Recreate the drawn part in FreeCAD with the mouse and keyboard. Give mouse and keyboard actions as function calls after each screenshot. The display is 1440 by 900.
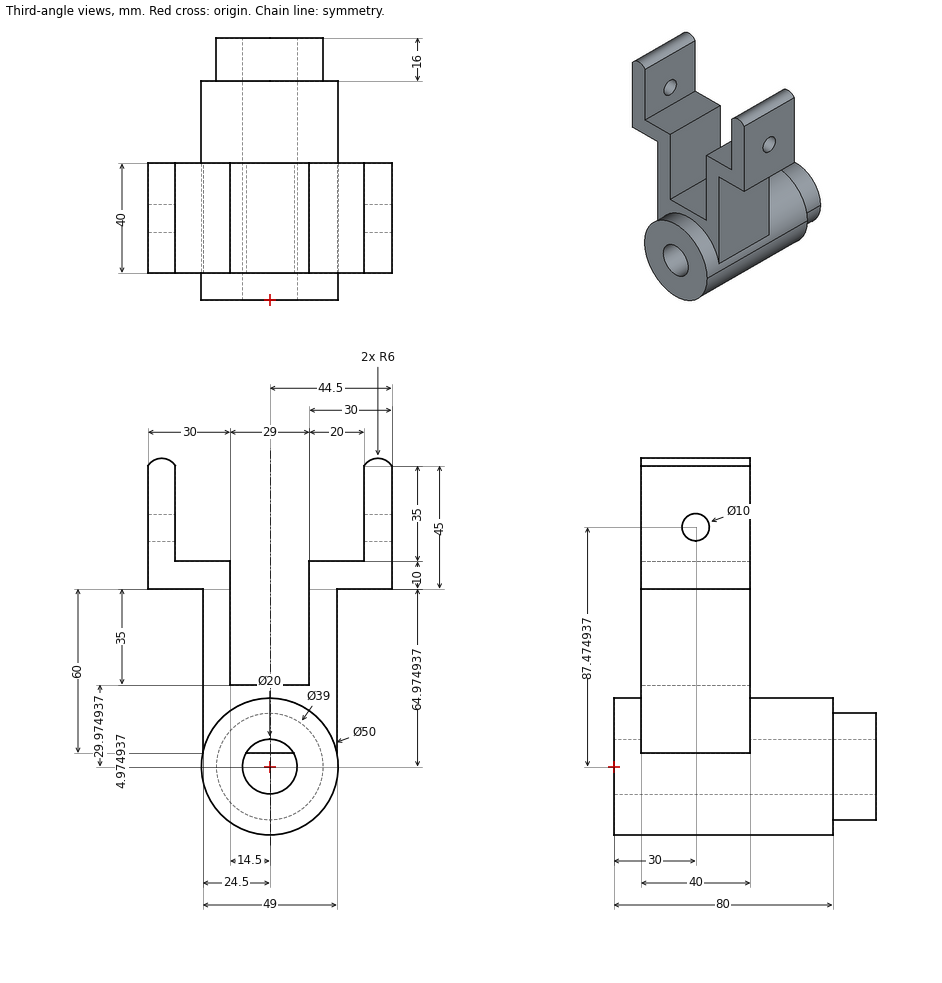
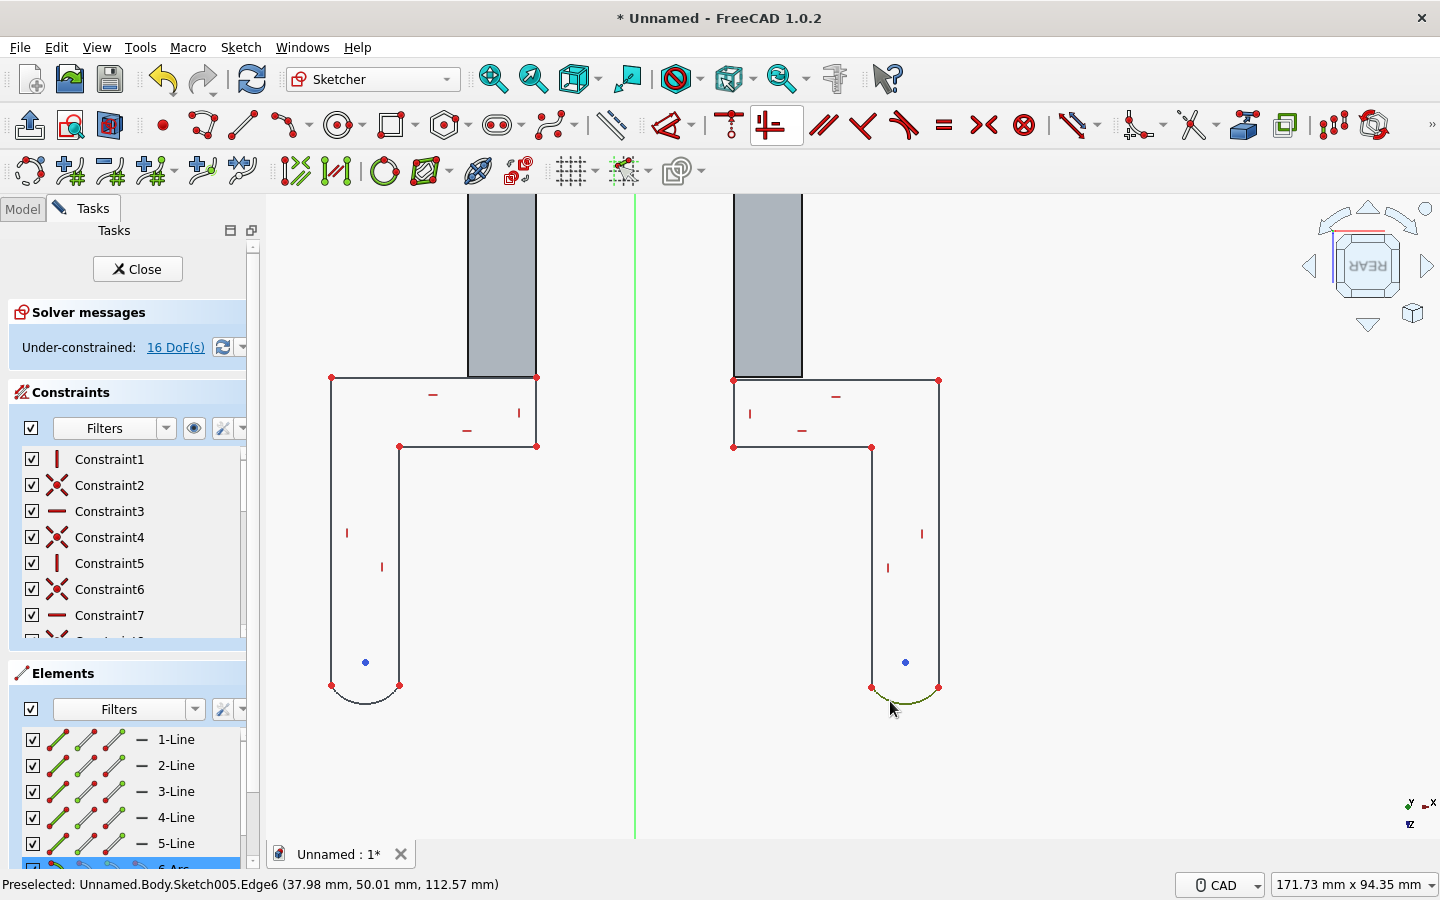
click(349, 701)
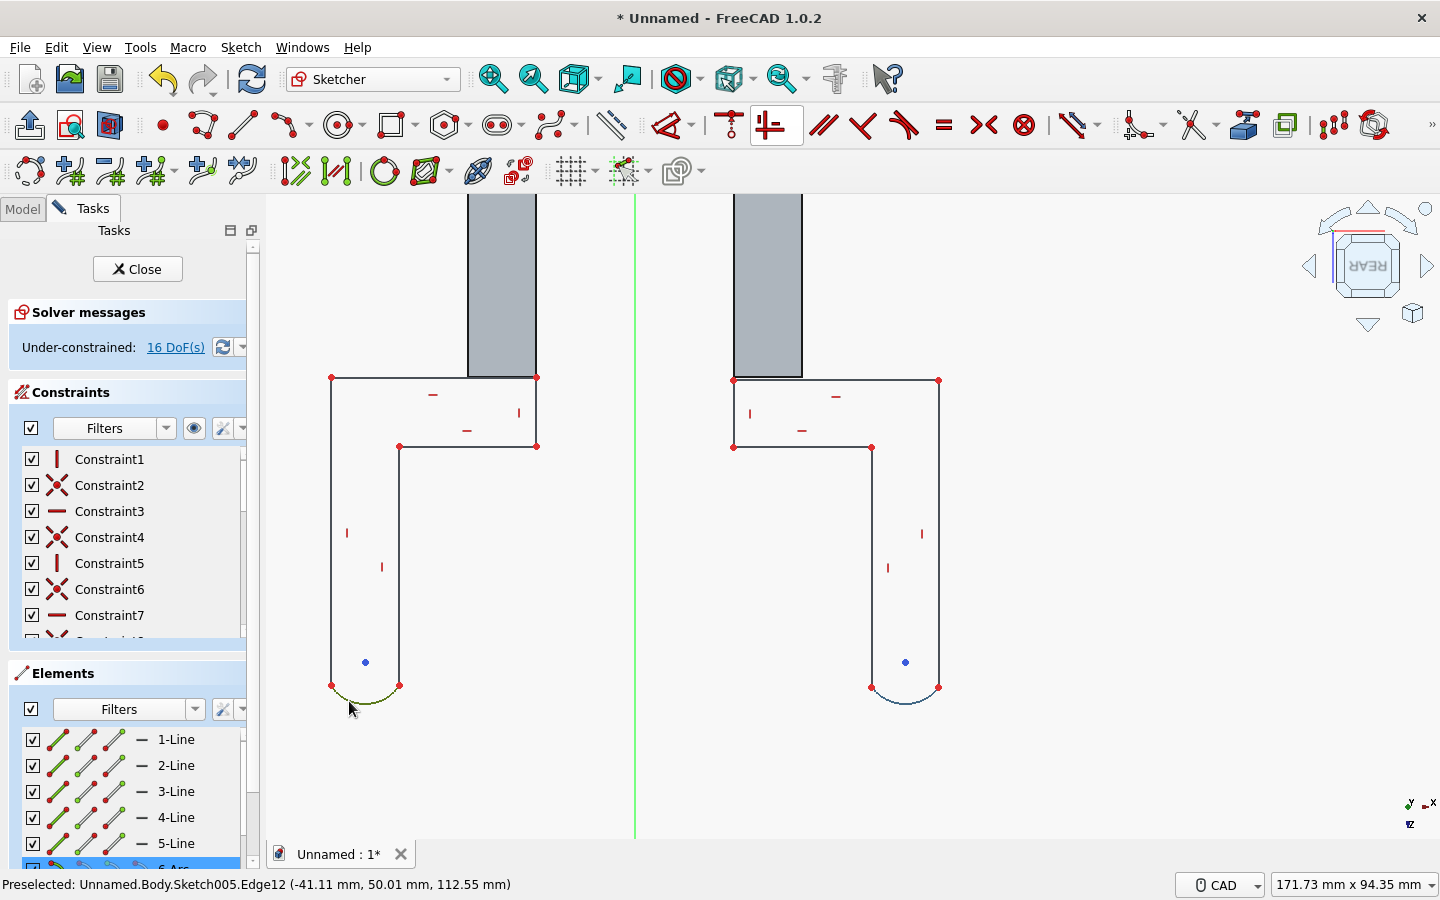
click(944, 126)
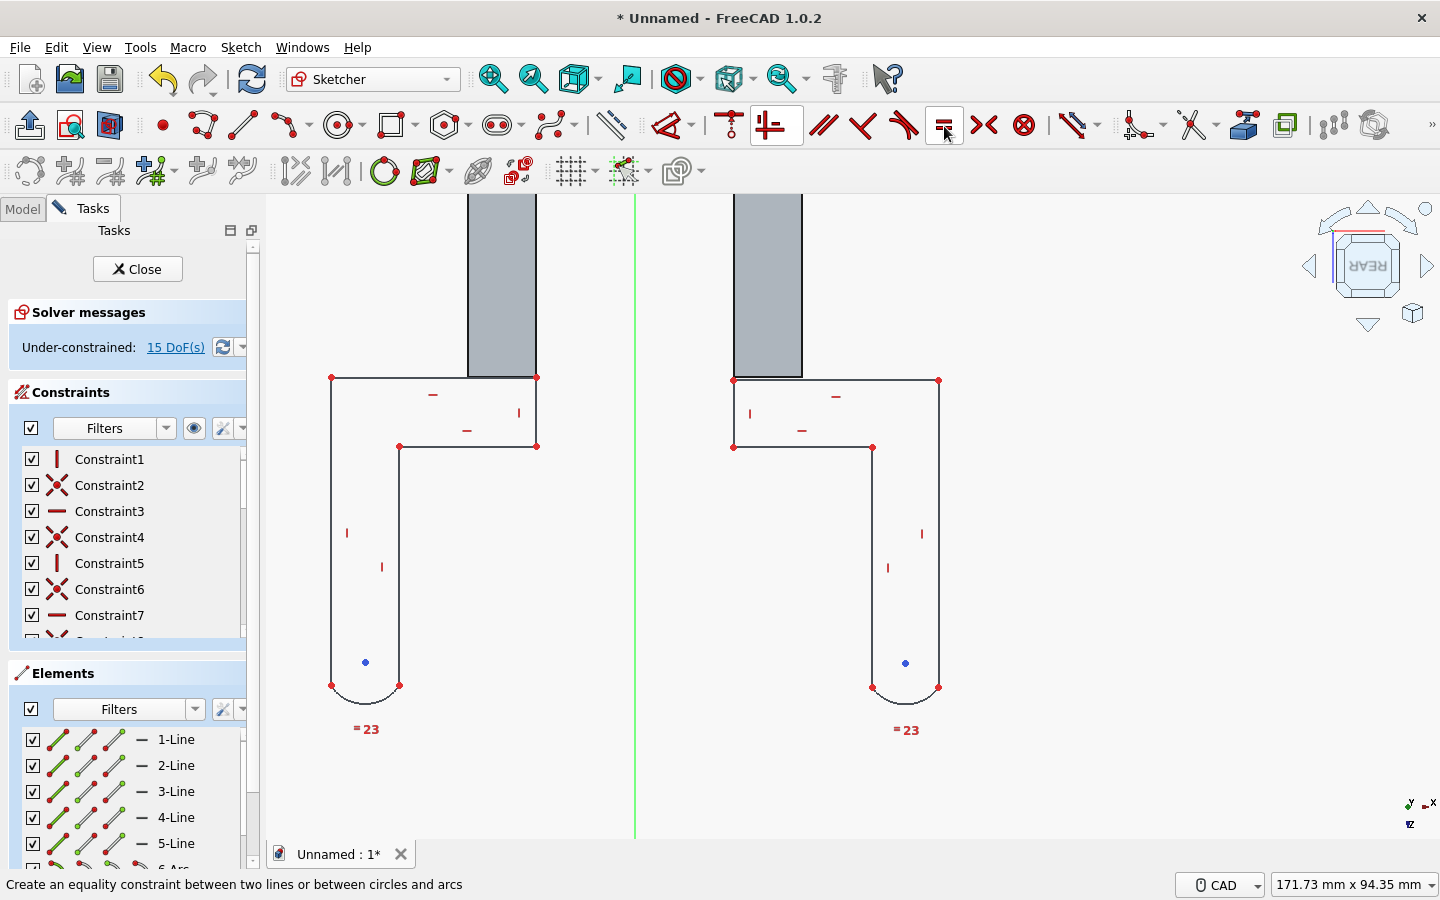
click(905, 663)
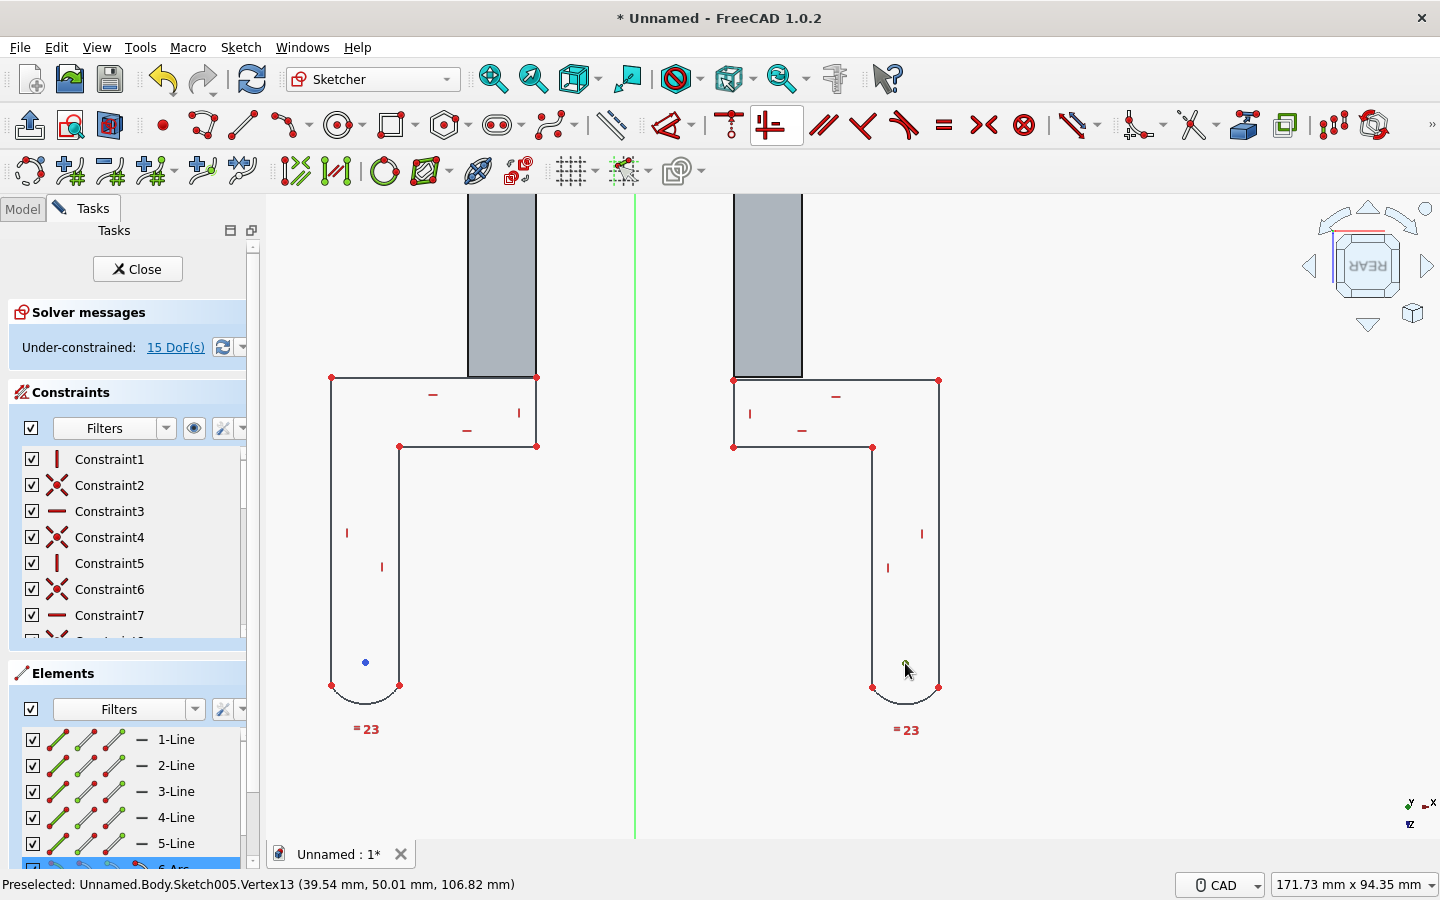
click(365, 663)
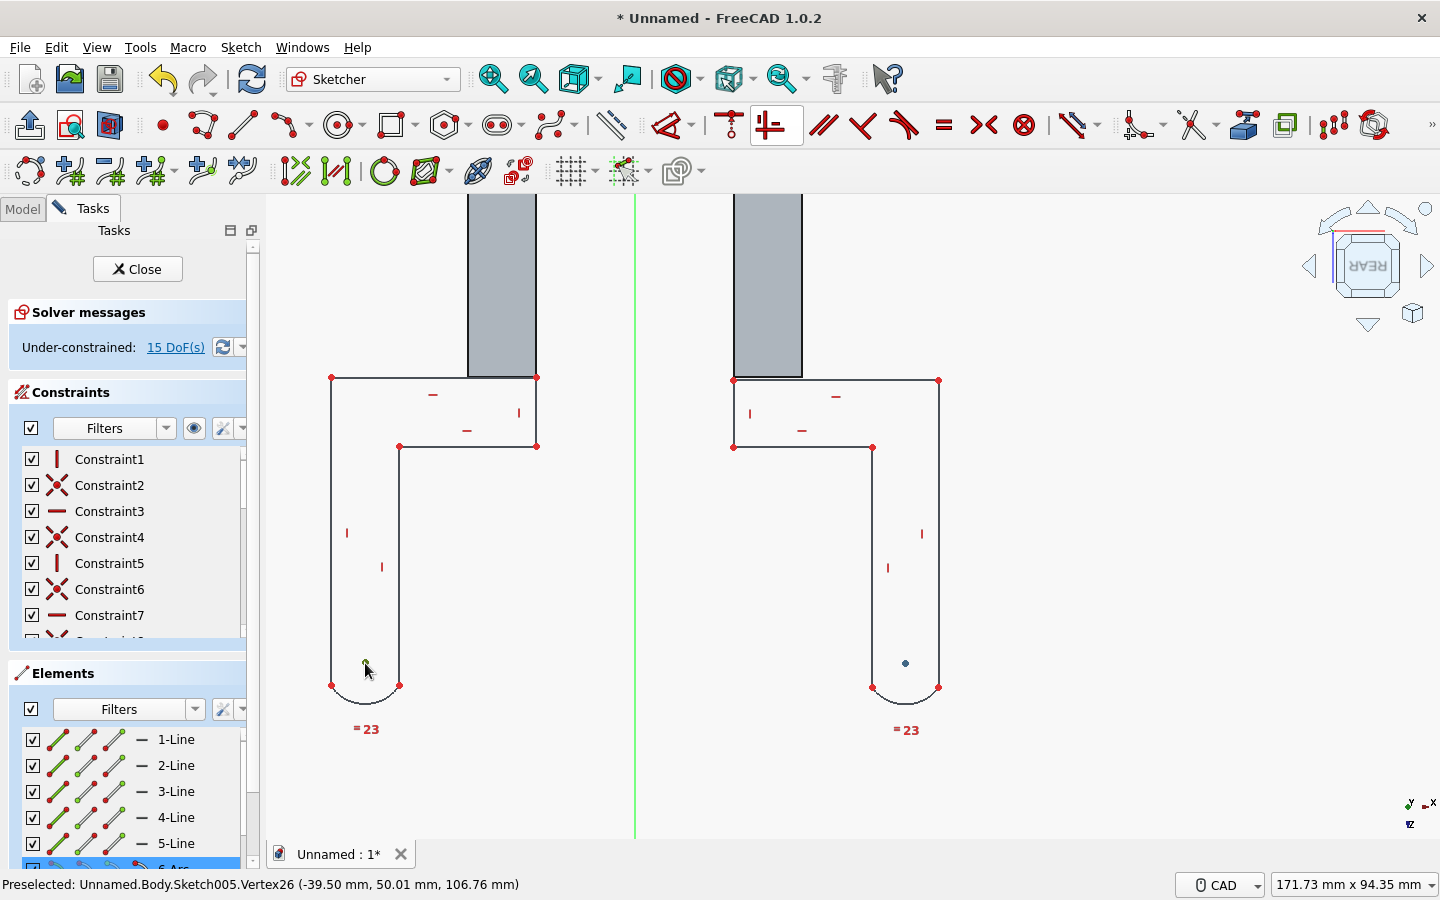
click(635, 769)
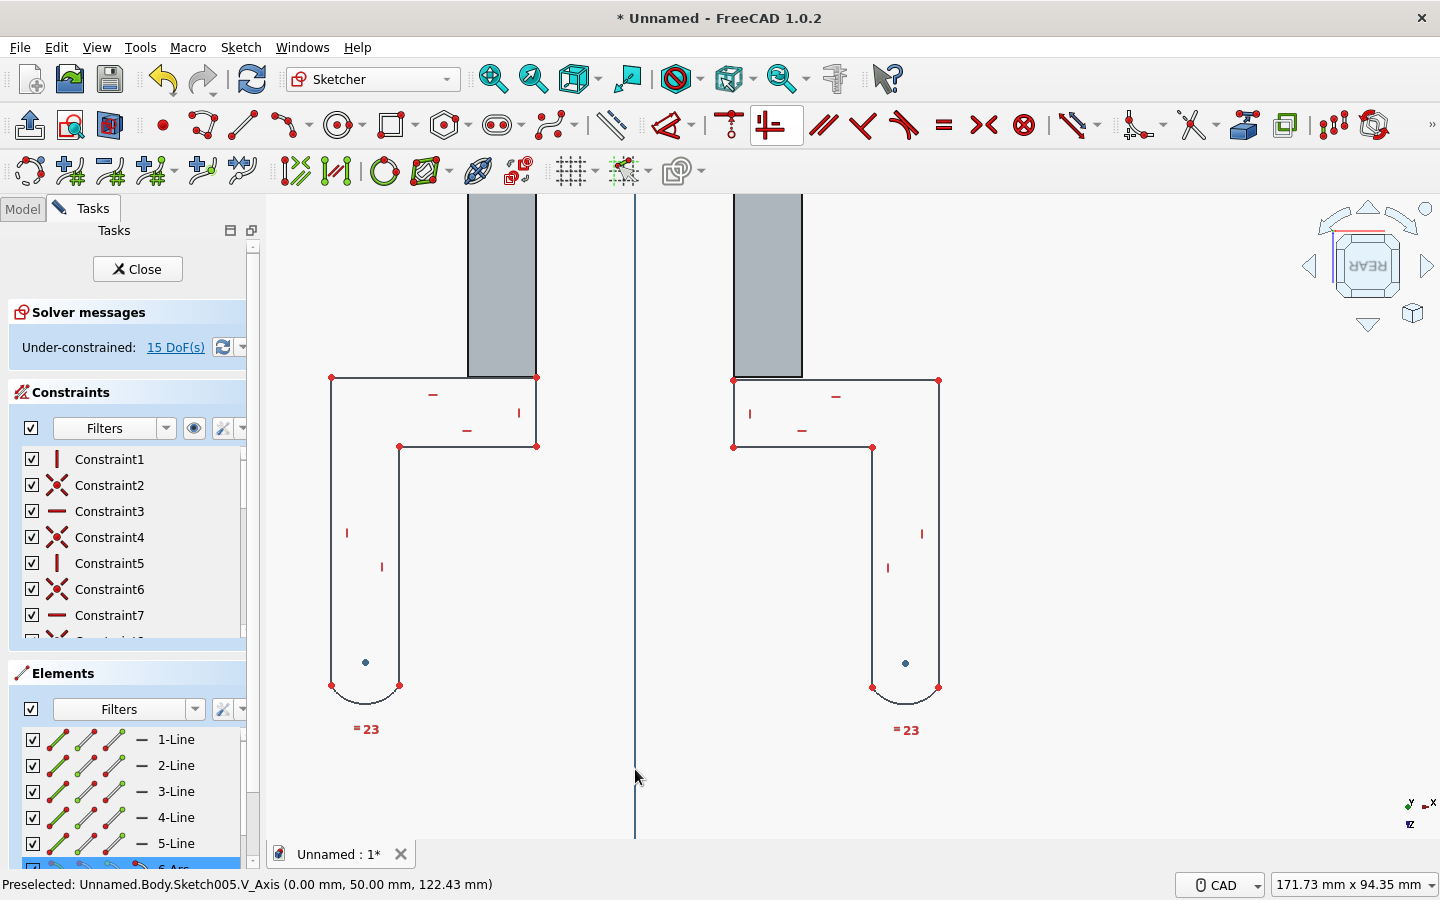
click(984, 126)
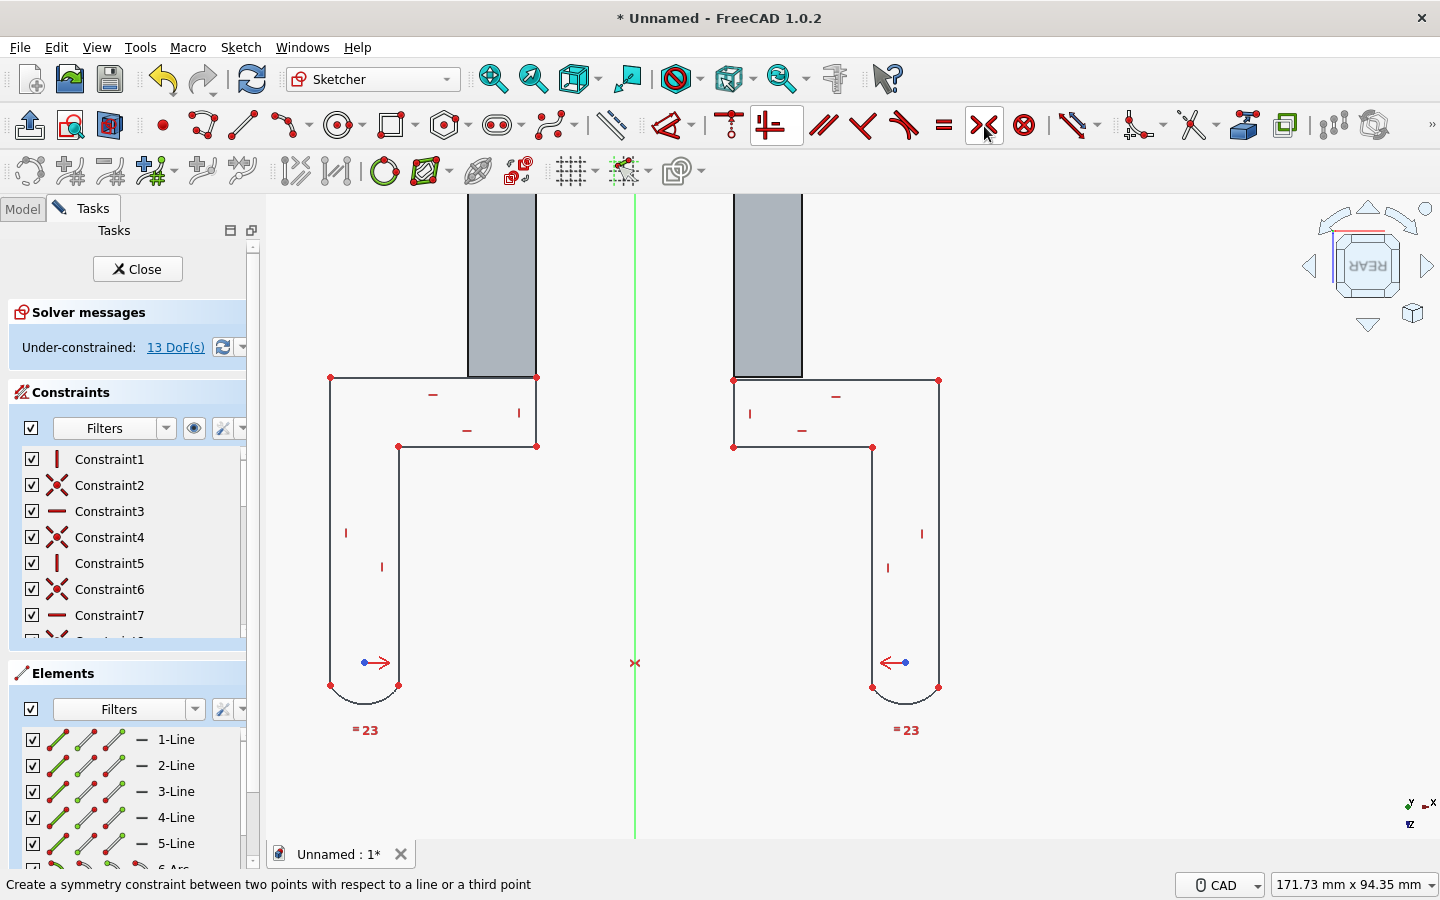
click(872, 447)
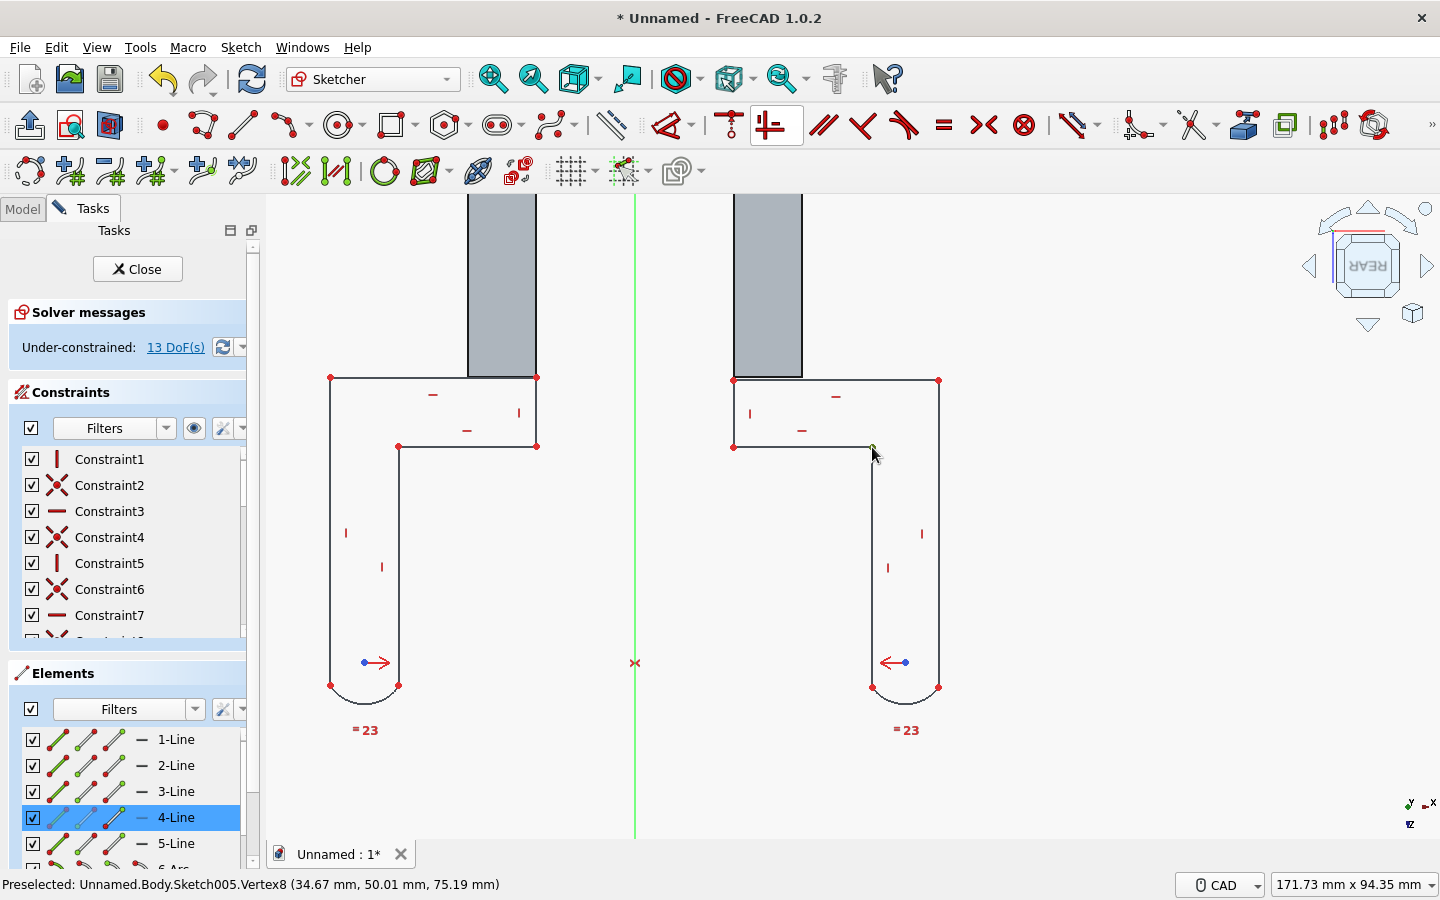
click(399, 447)